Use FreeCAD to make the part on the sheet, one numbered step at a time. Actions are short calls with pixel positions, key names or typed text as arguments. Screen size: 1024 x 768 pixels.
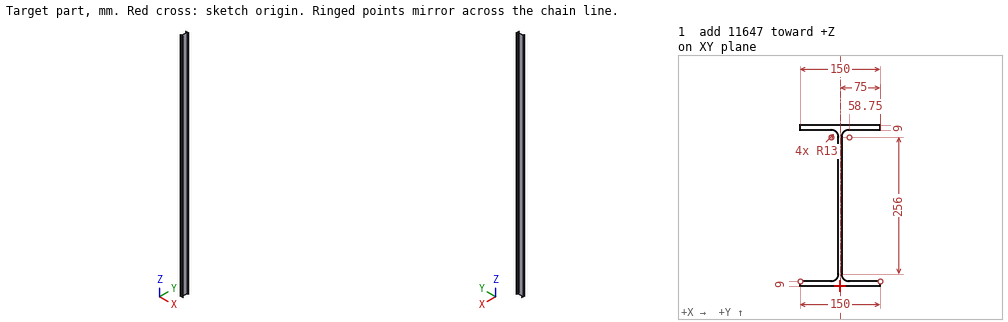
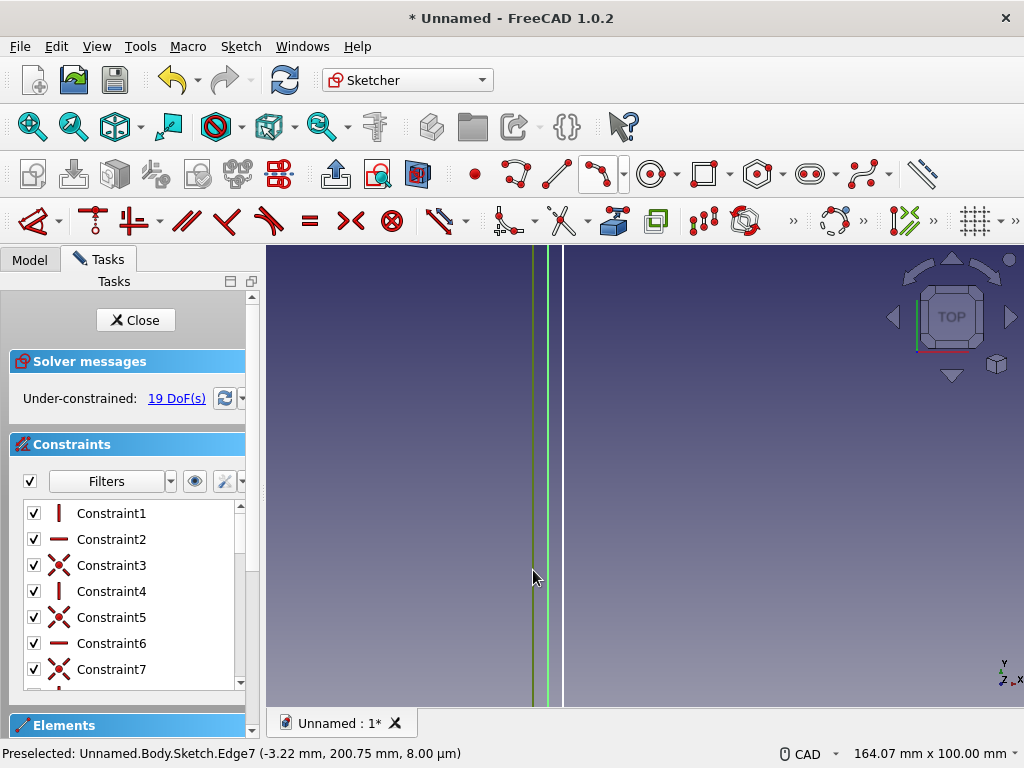
scroll(584, 393, down, 8)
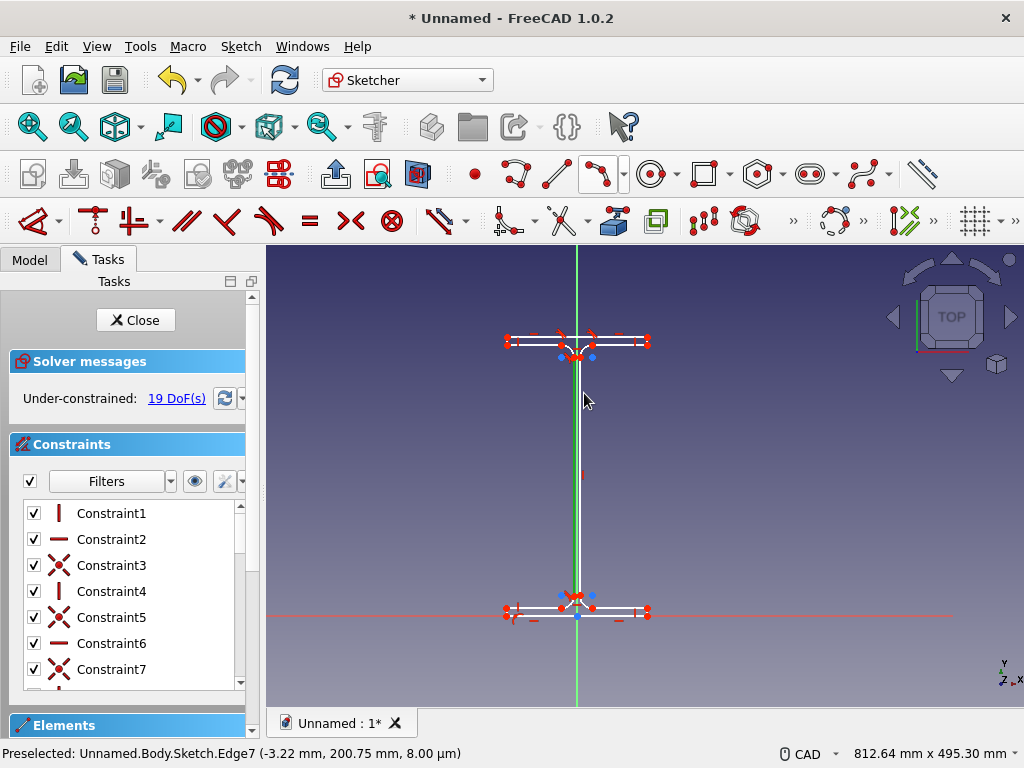
scroll(573, 352, up, 6)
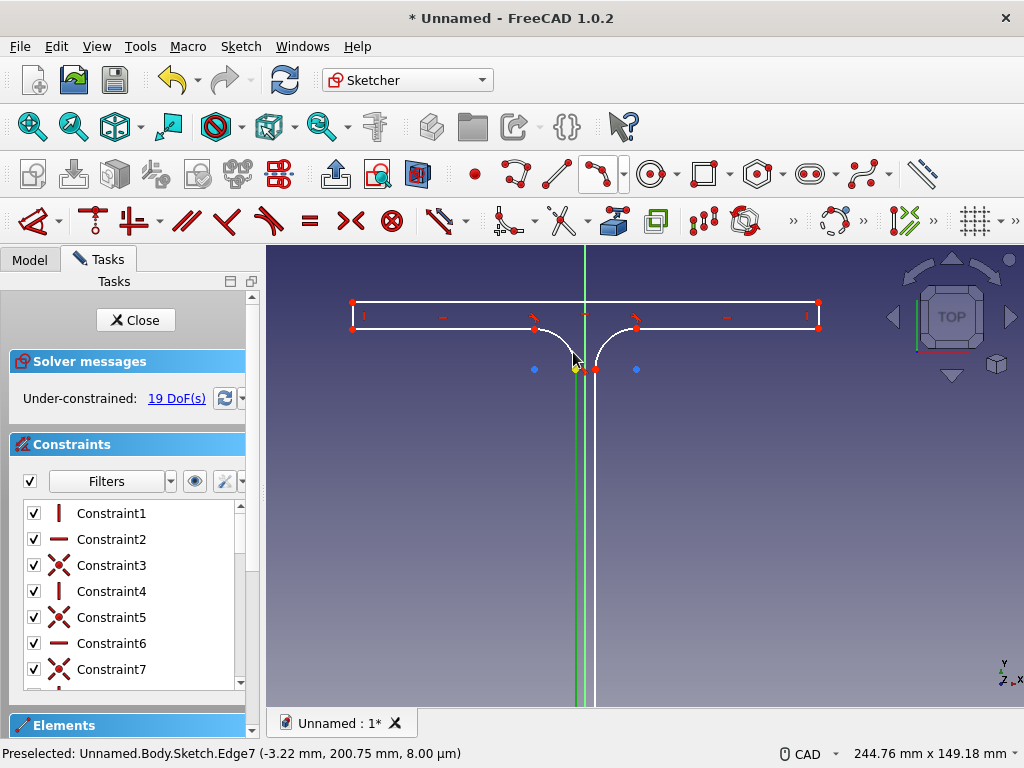
click(571, 351)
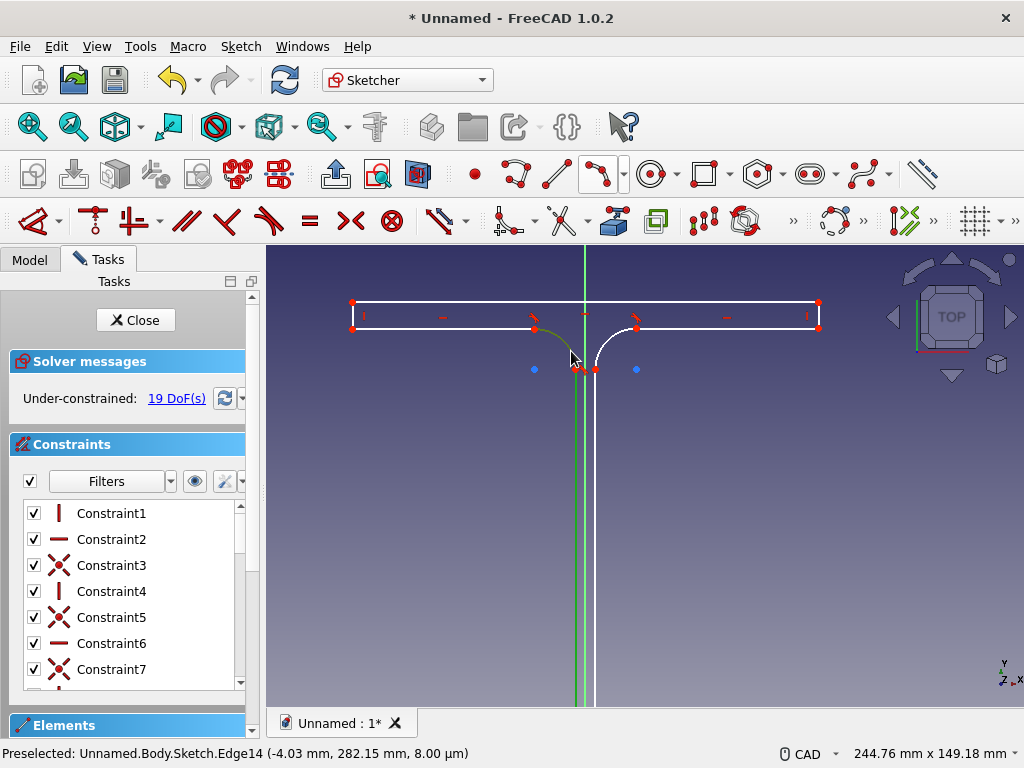
key(t)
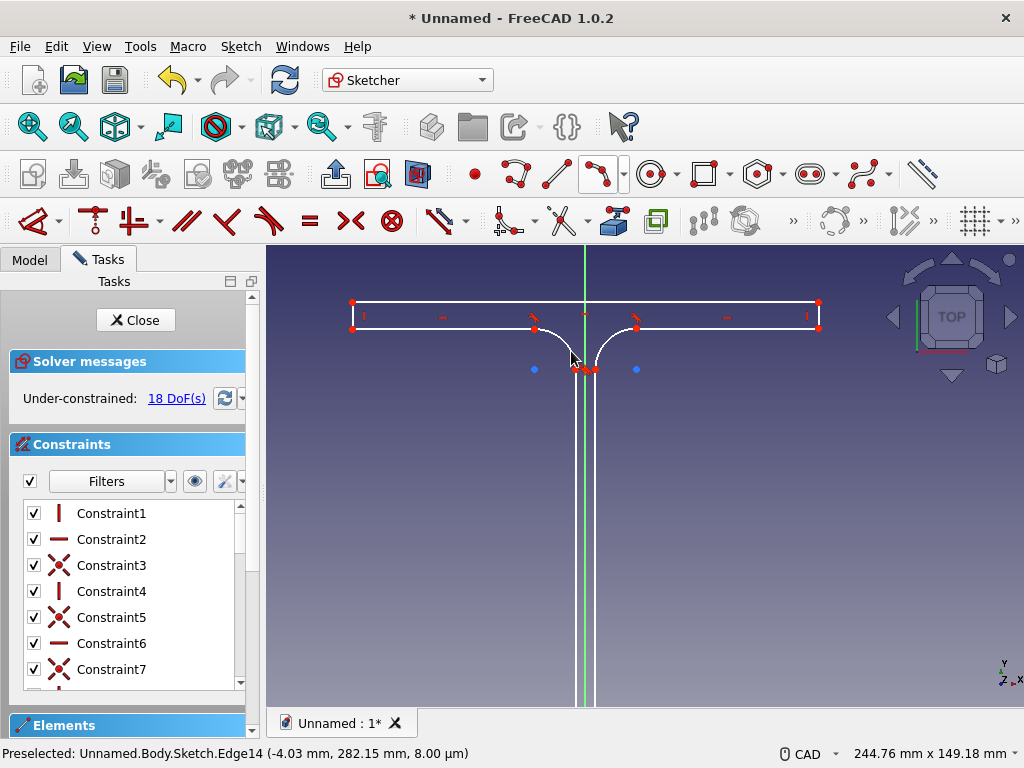
scroll(576, 607, up, 2)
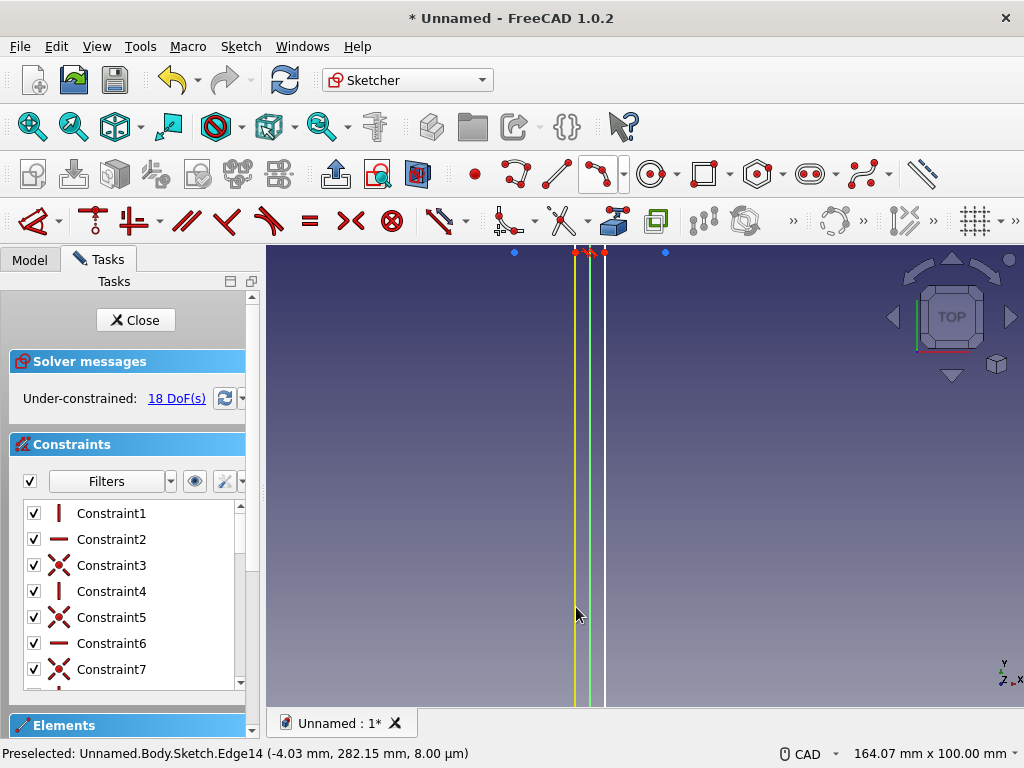
click(575, 607)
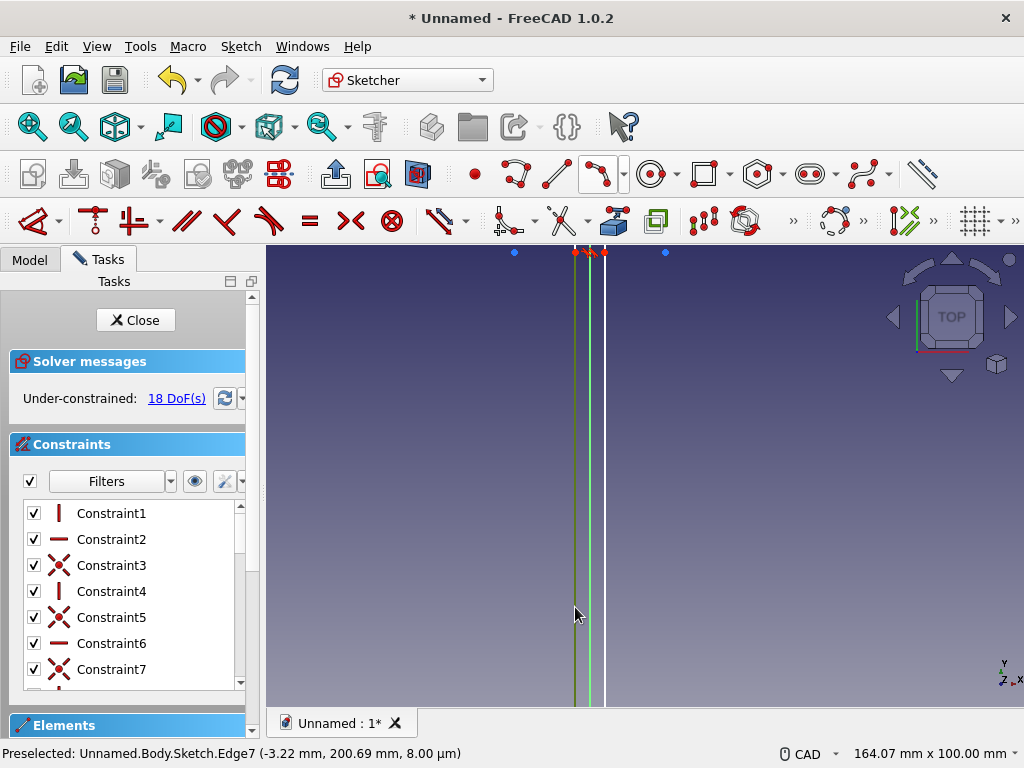
scroll(573, 383, down, 8)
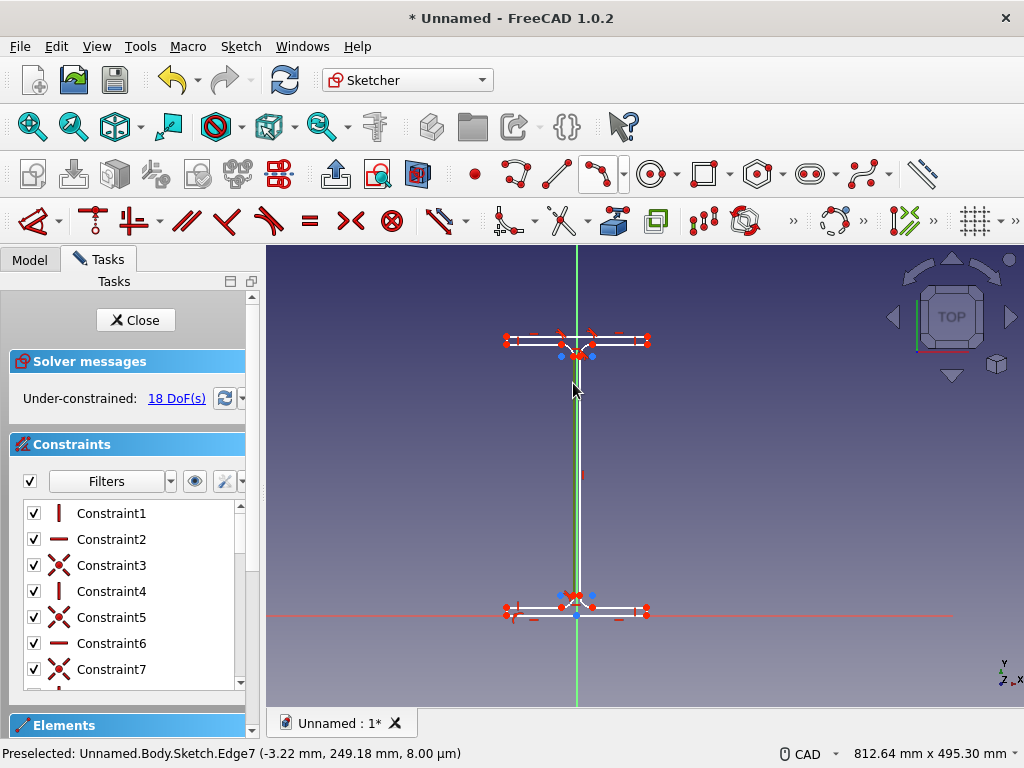
scroll(567, 606, up, 5)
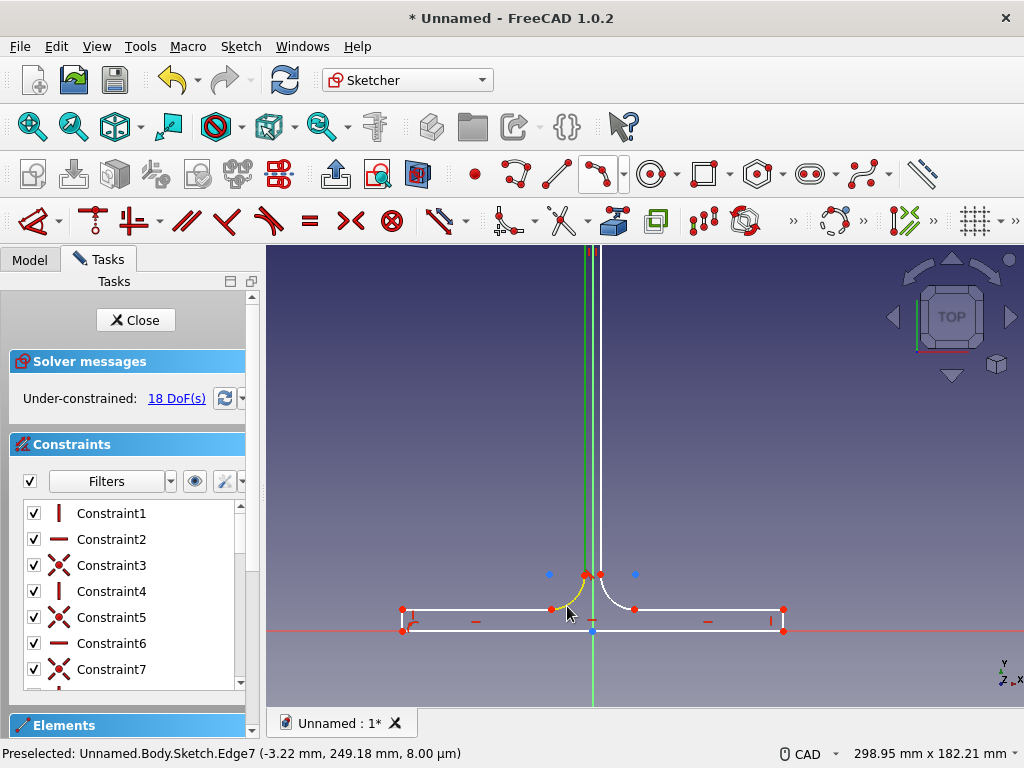
click(566, 606)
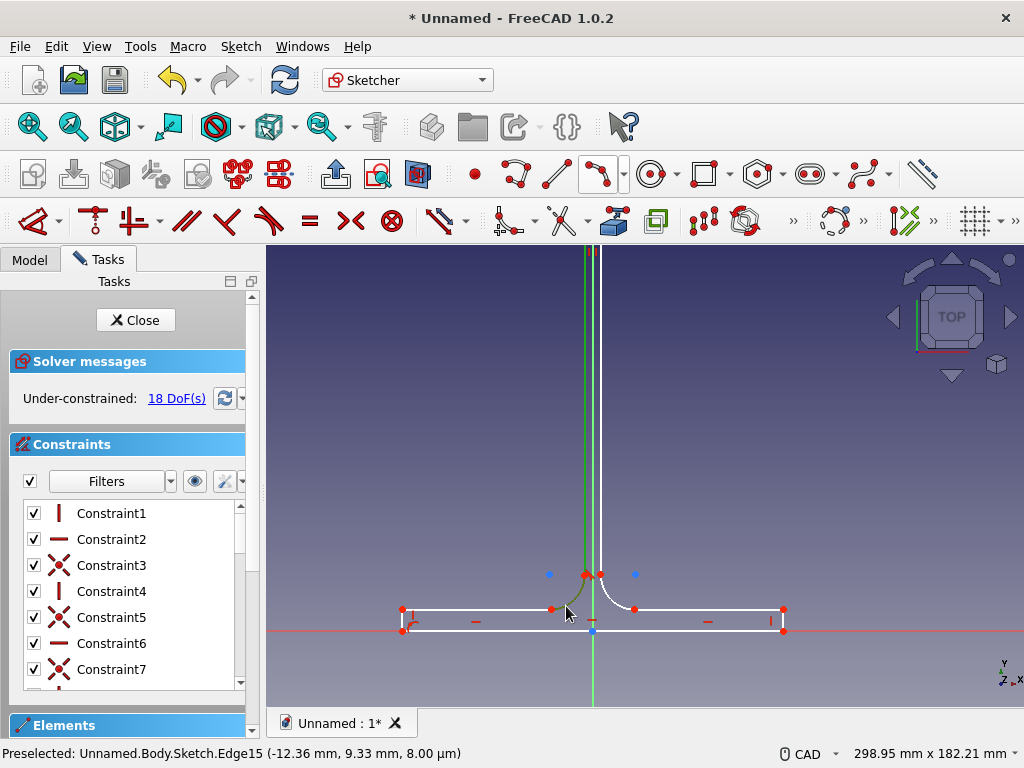
key(t)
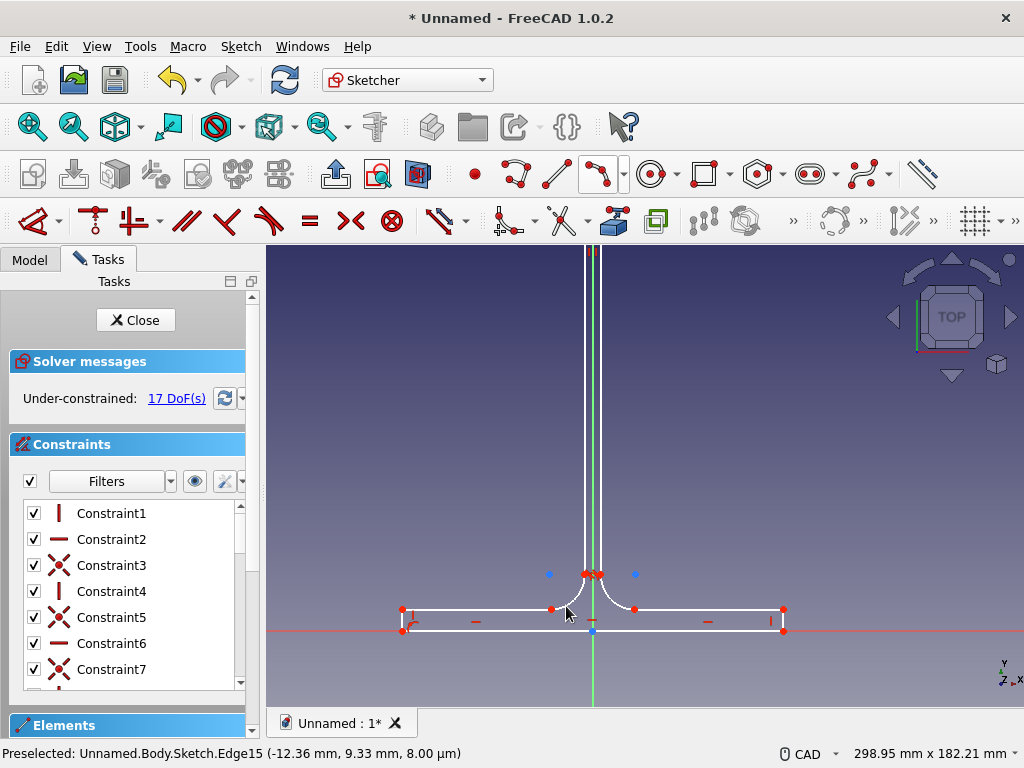
click(507, 610)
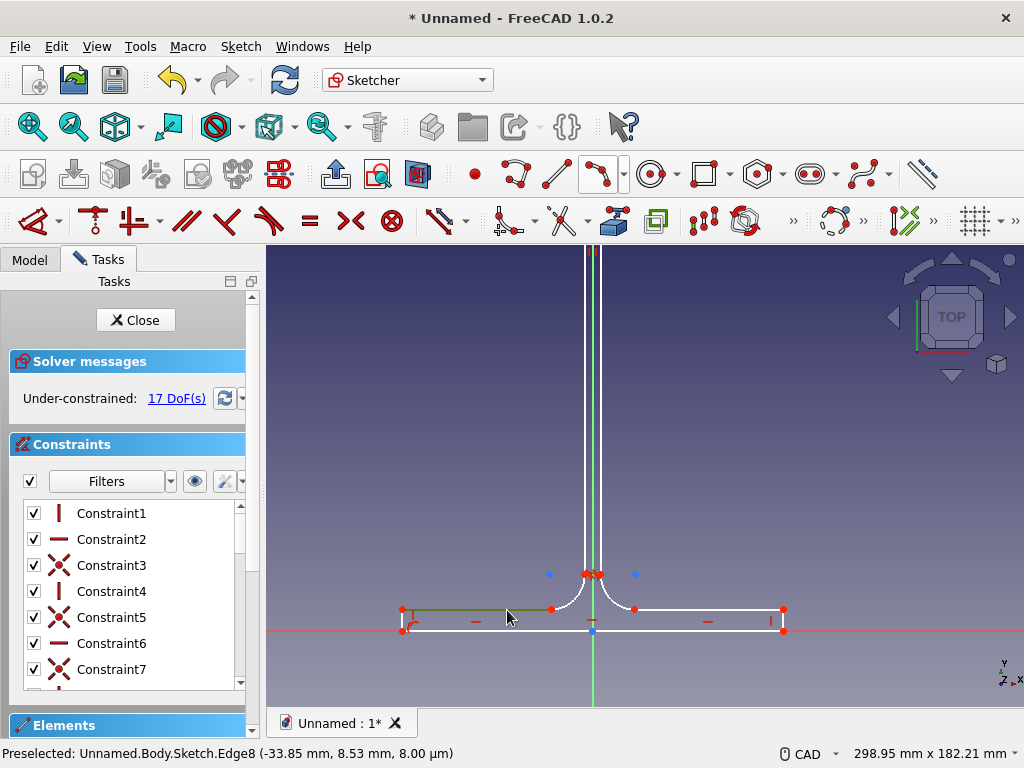
click(567, 606)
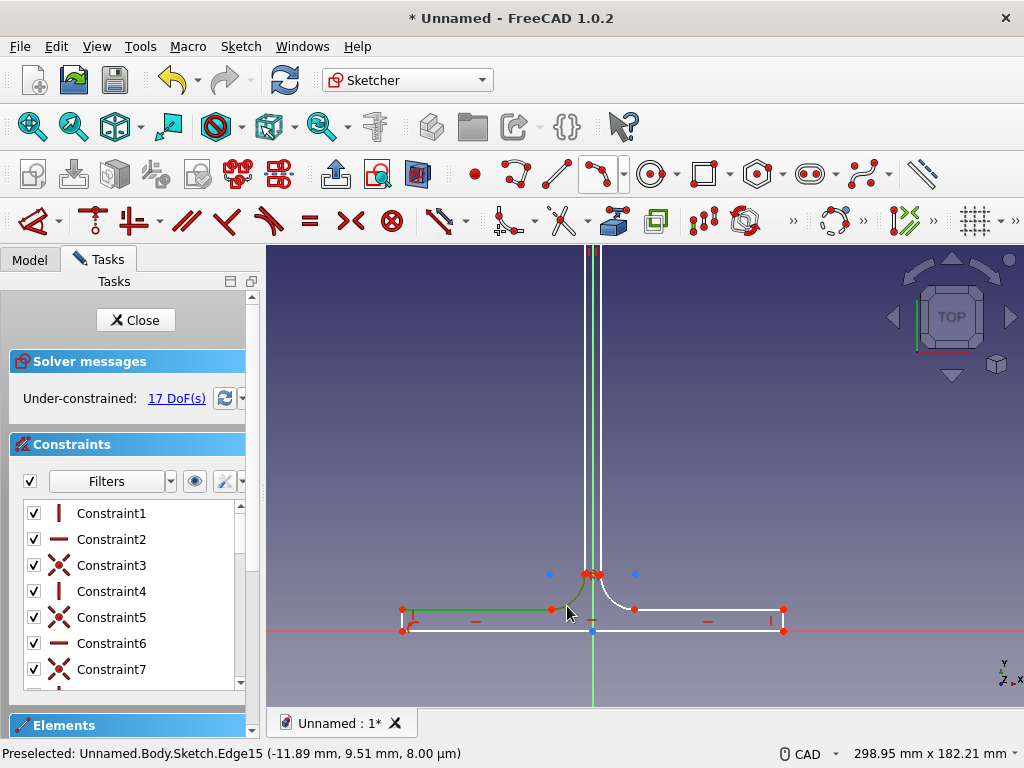
key(t)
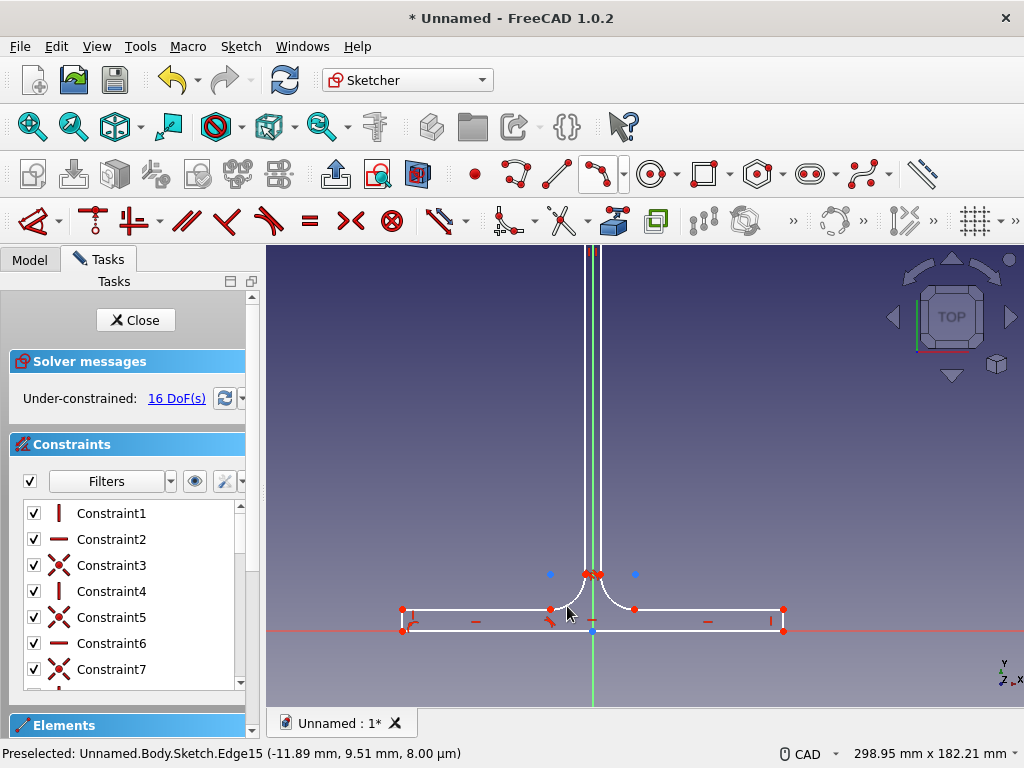
click(739, 610)